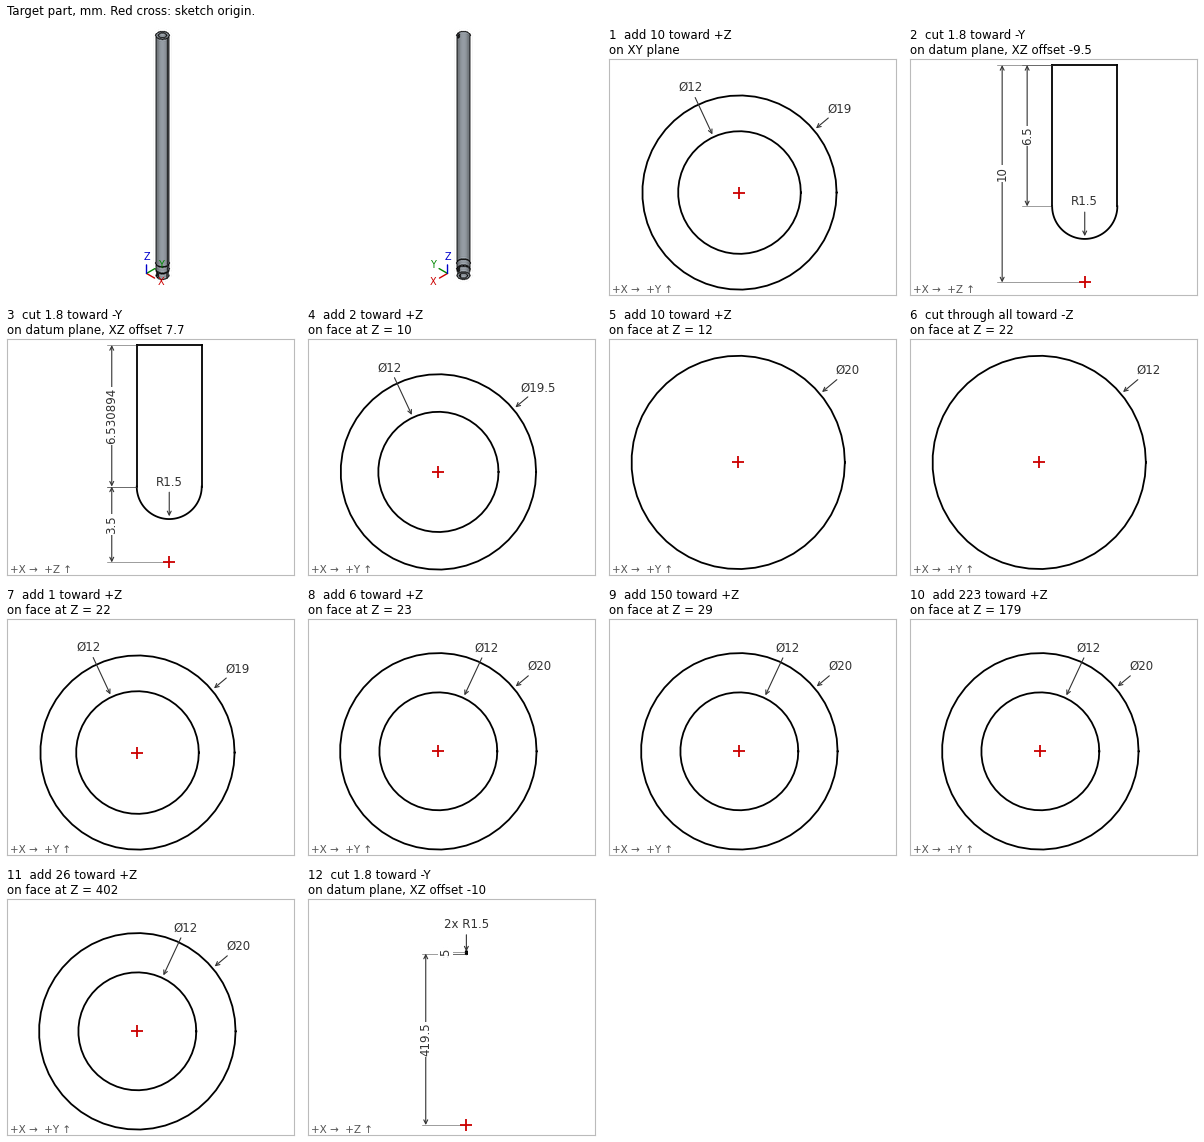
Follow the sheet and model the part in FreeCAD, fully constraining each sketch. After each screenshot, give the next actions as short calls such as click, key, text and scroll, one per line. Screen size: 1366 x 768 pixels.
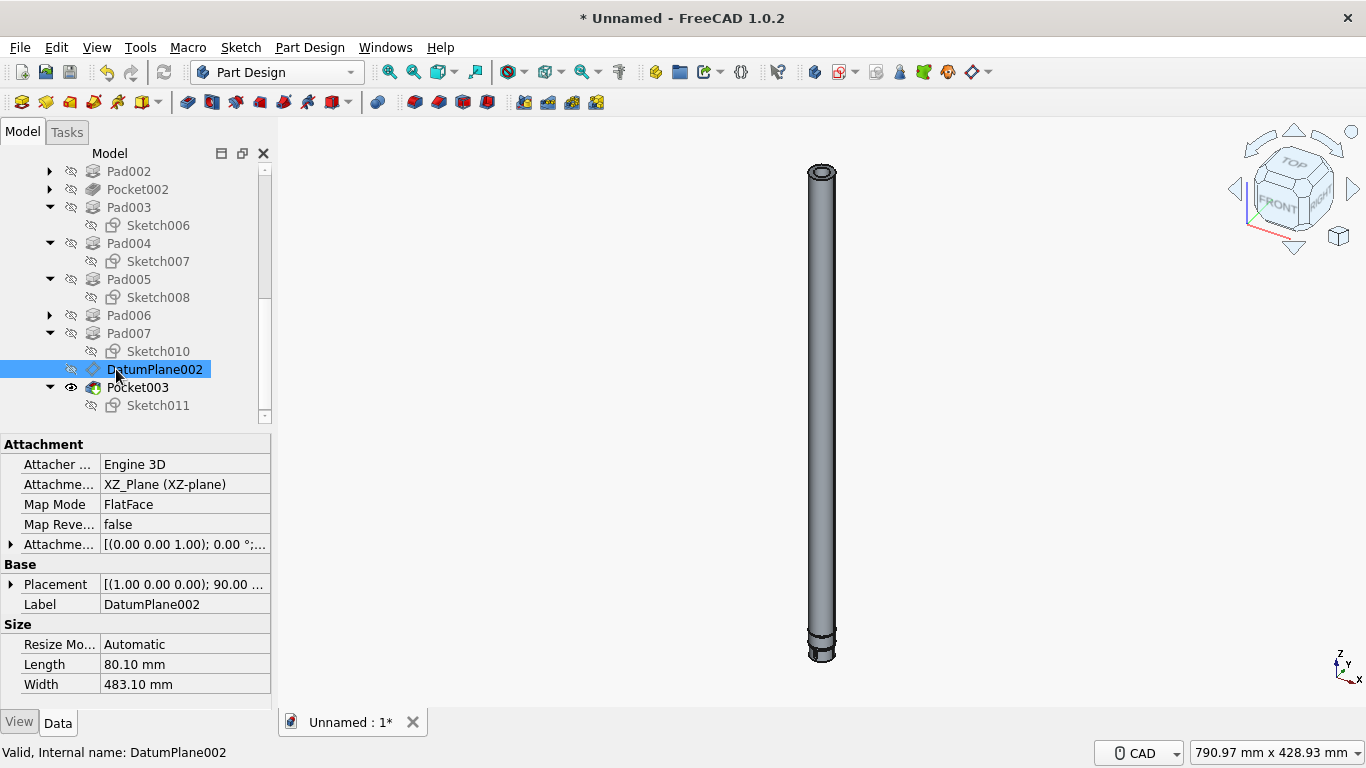
key(0)